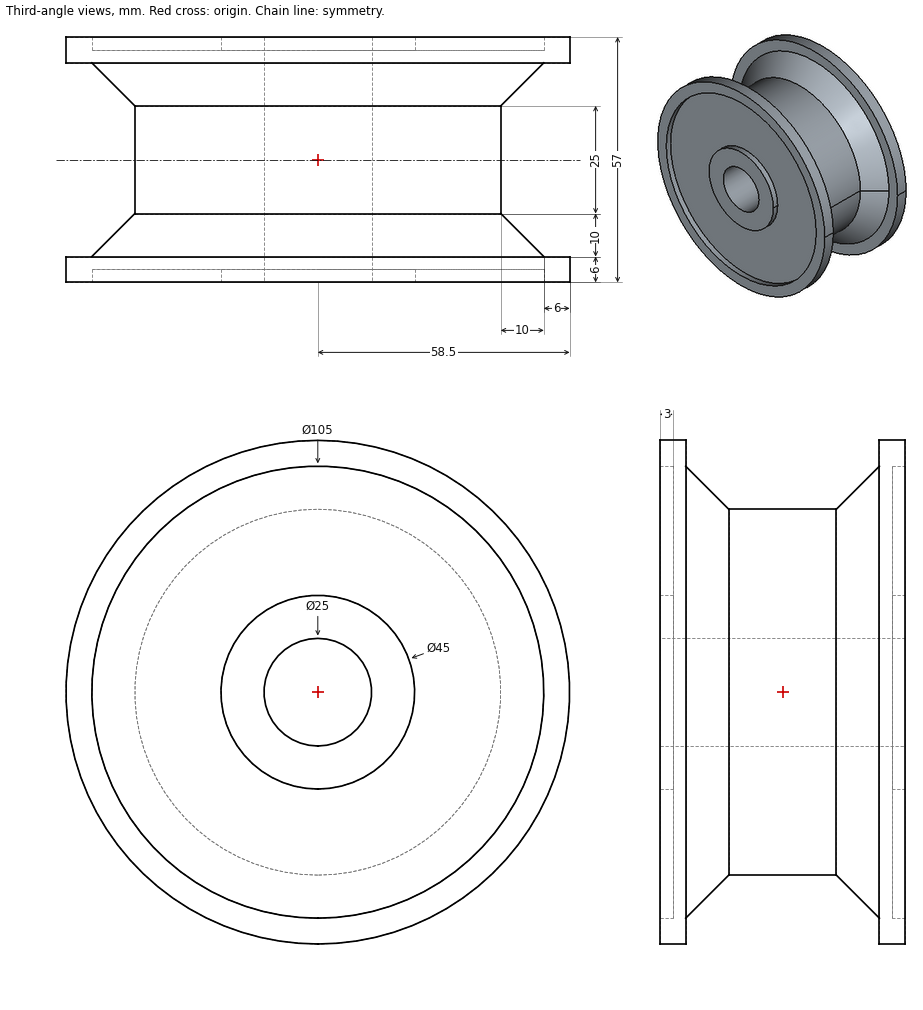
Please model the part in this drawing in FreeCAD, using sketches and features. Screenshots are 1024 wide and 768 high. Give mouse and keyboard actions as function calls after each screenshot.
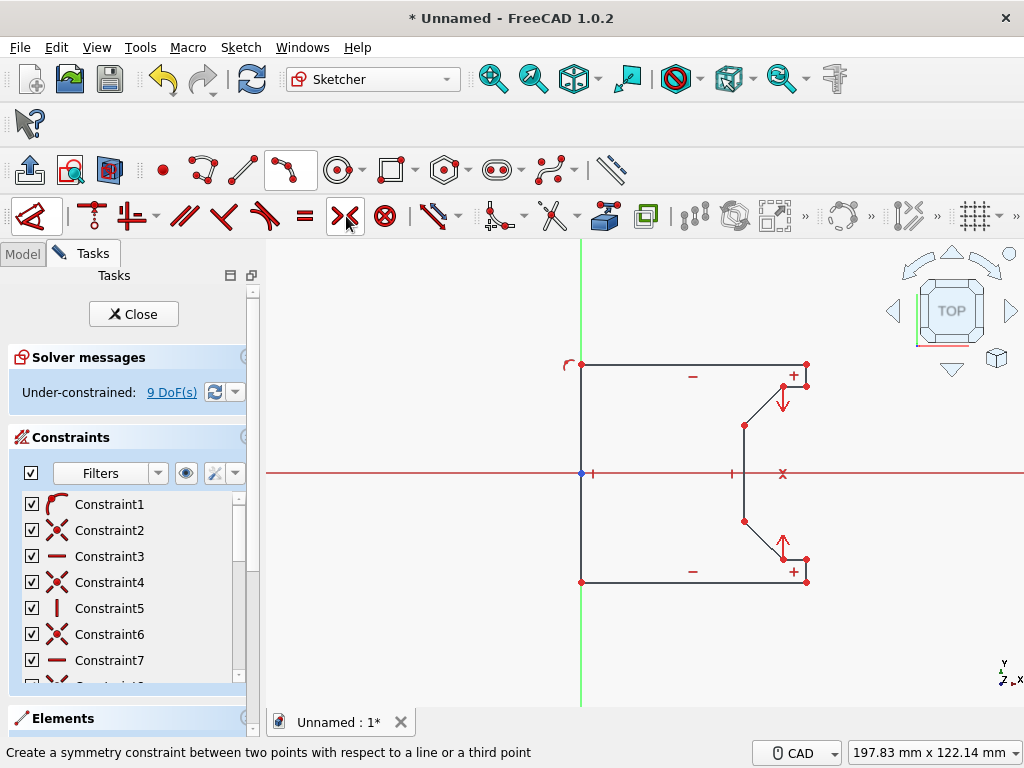
click(806, 583)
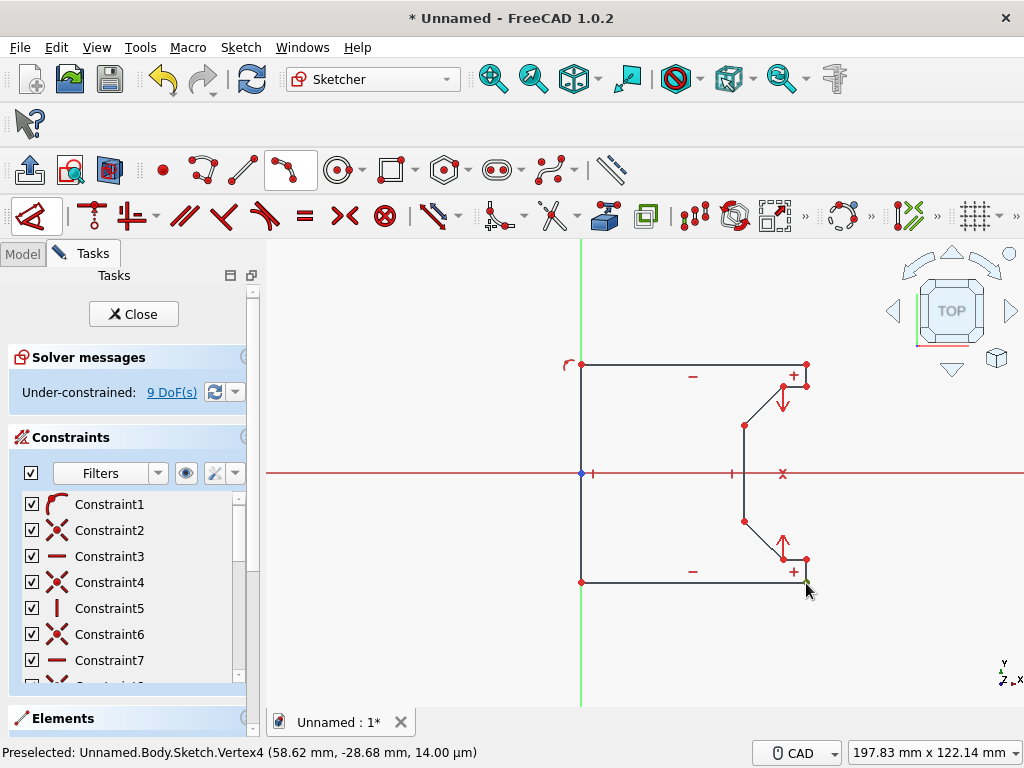
click(806, 365)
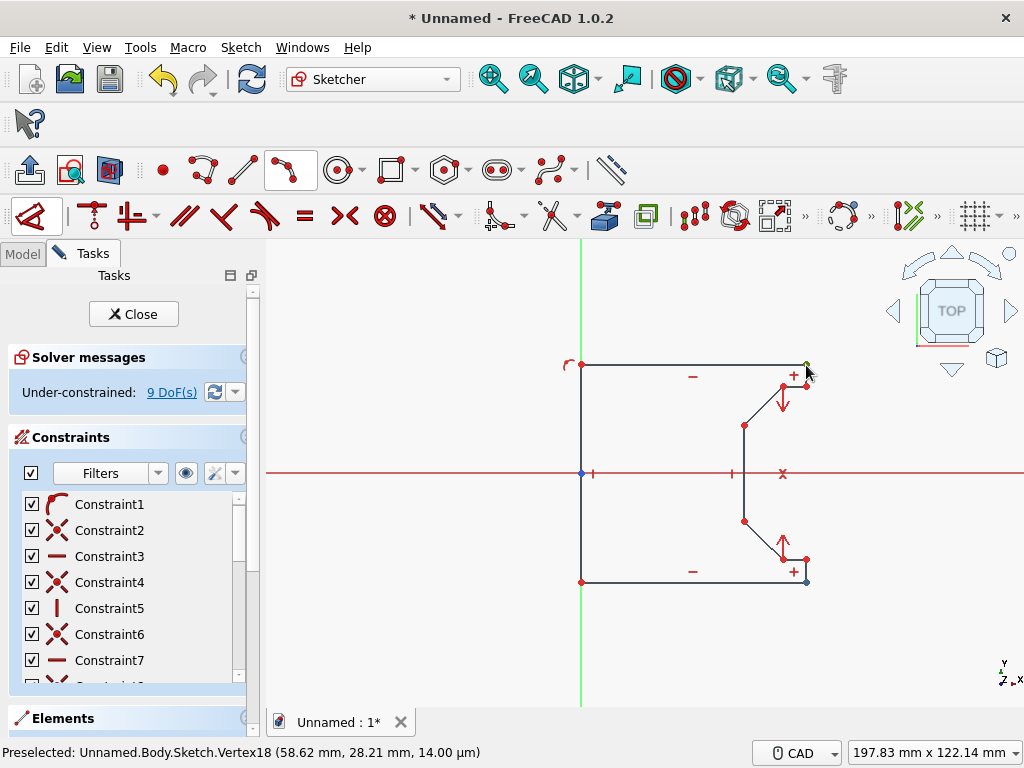
click(334, 473)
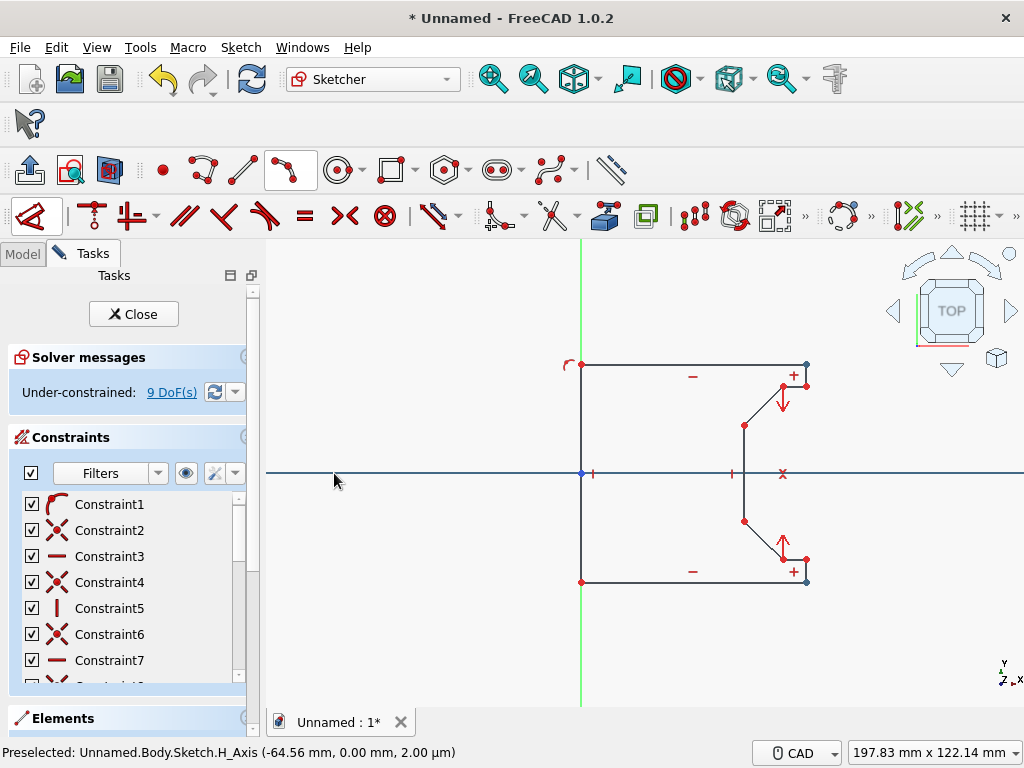
click(346, 216)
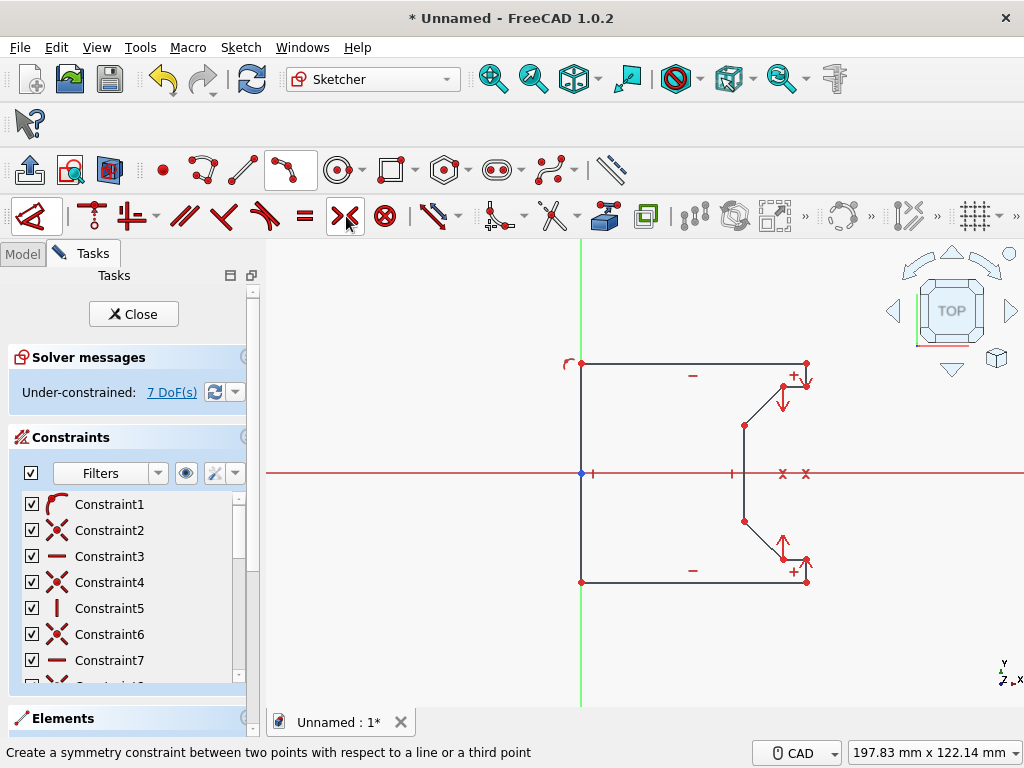
click(30, 216)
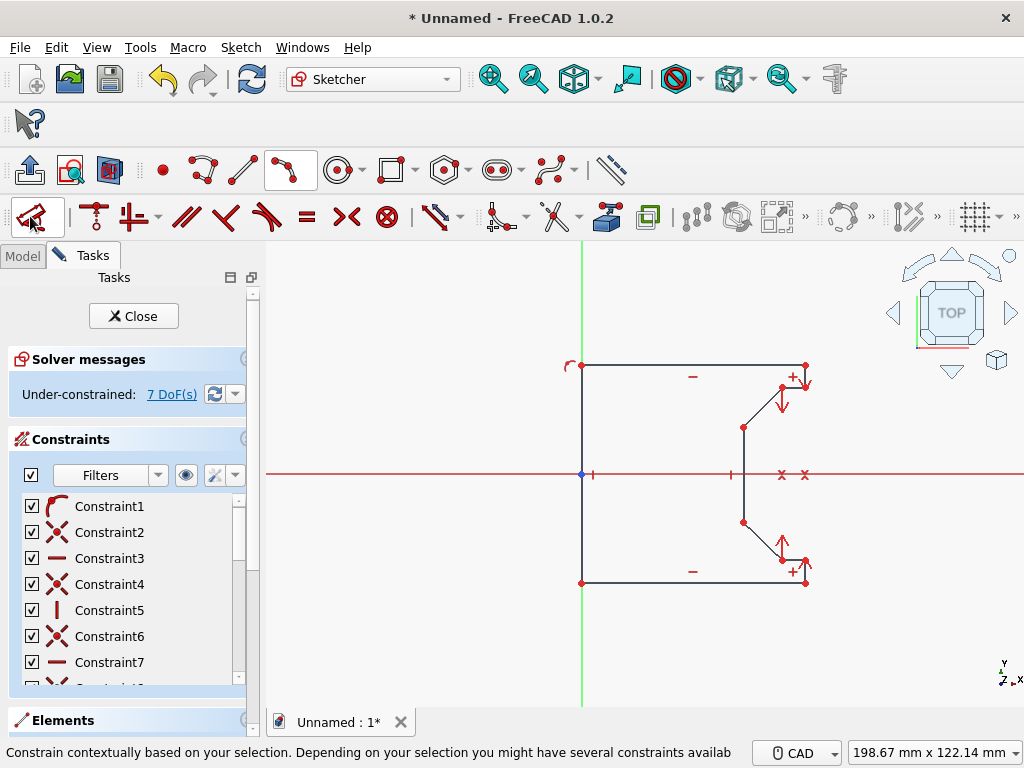
scroll(805, 574, up, 3)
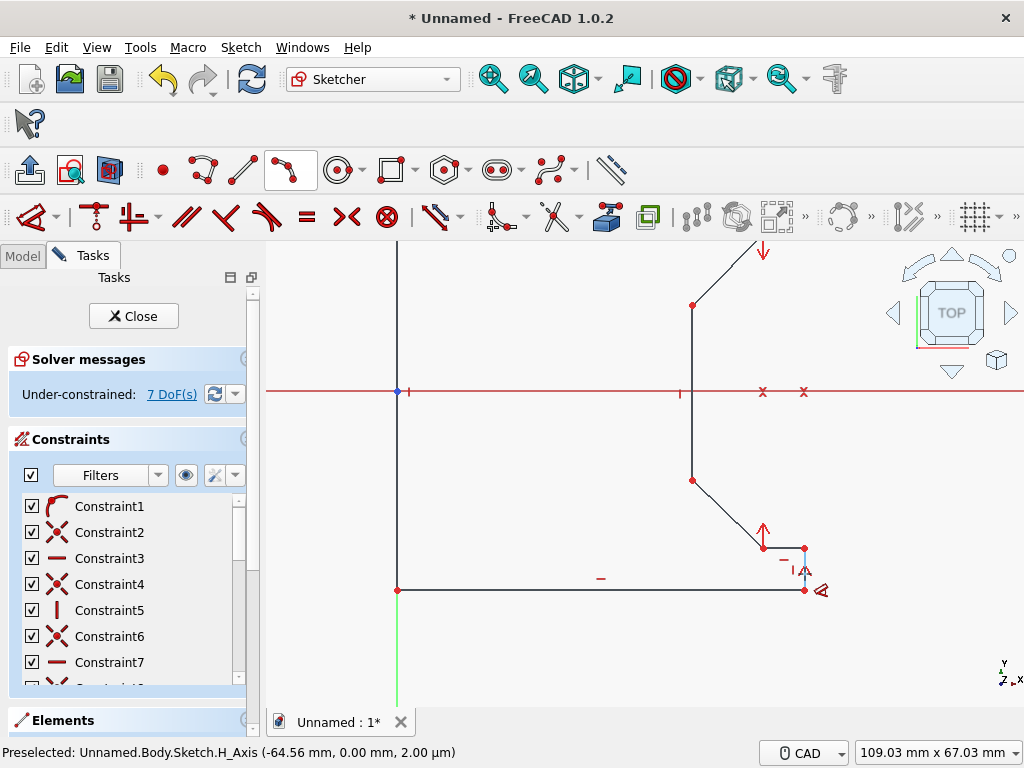
click(805, 573)
click(839, 569)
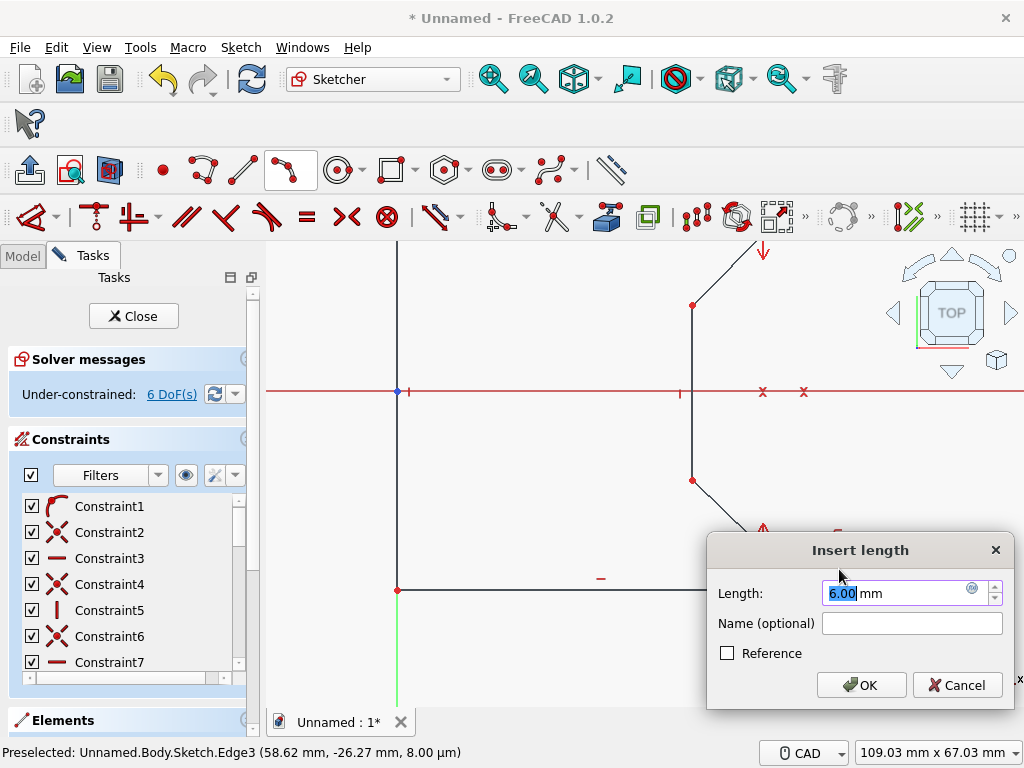
text(6)
key(Return)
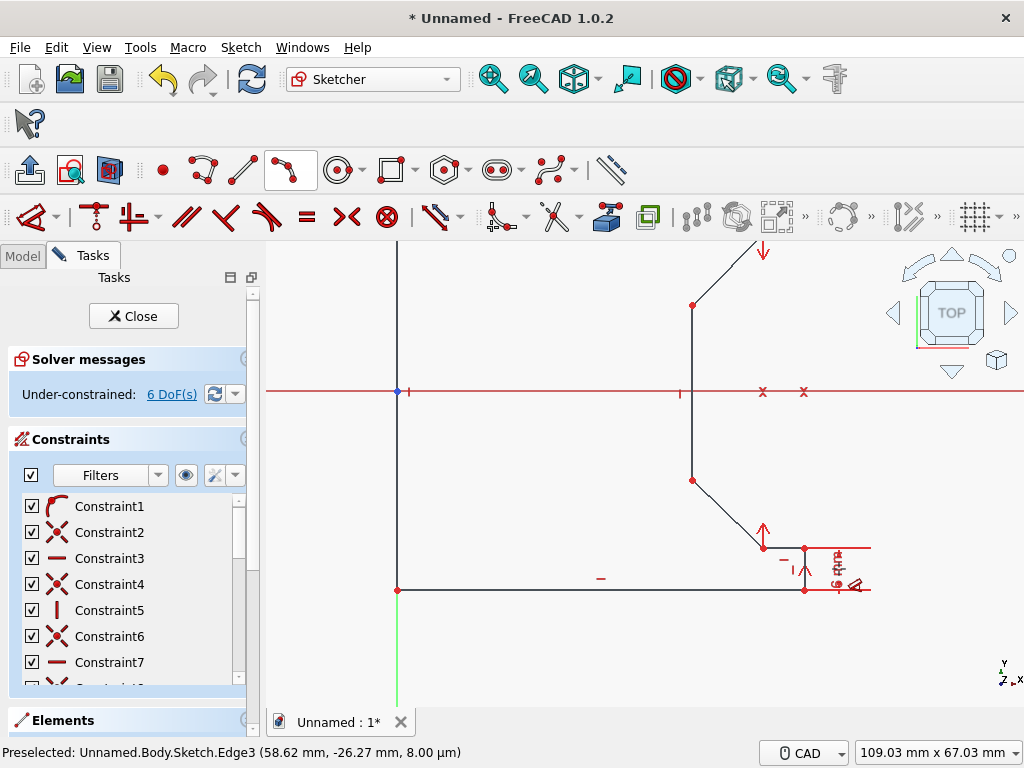
click(792, 548)
click(784, 514)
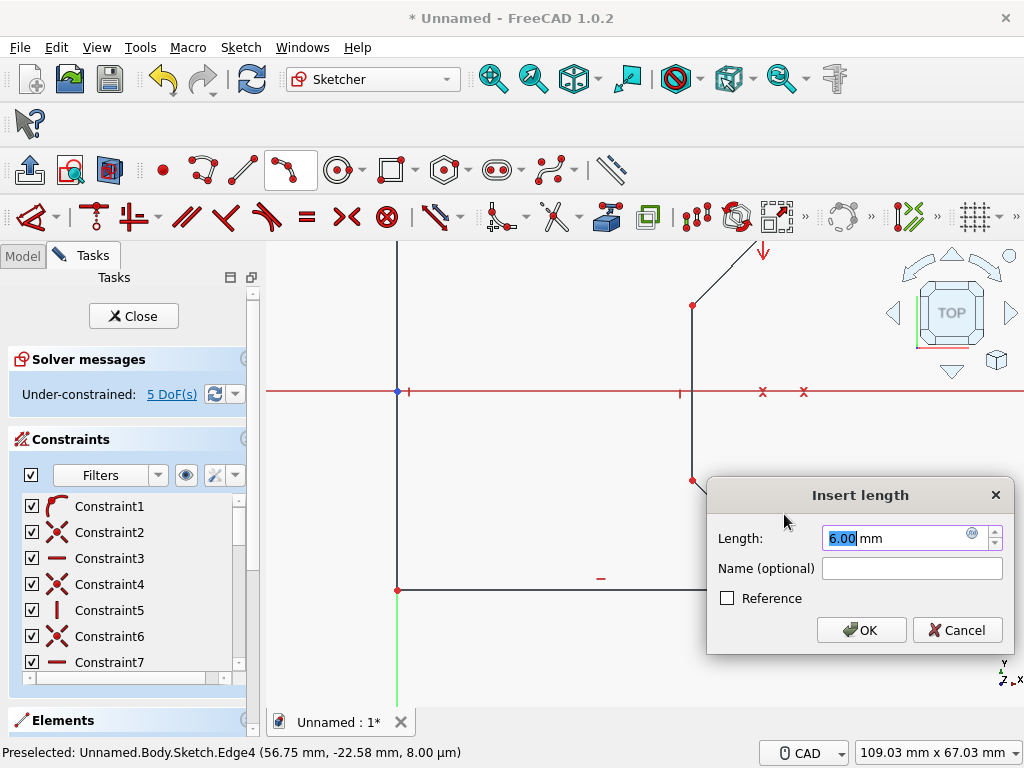
text(6)
key(Return)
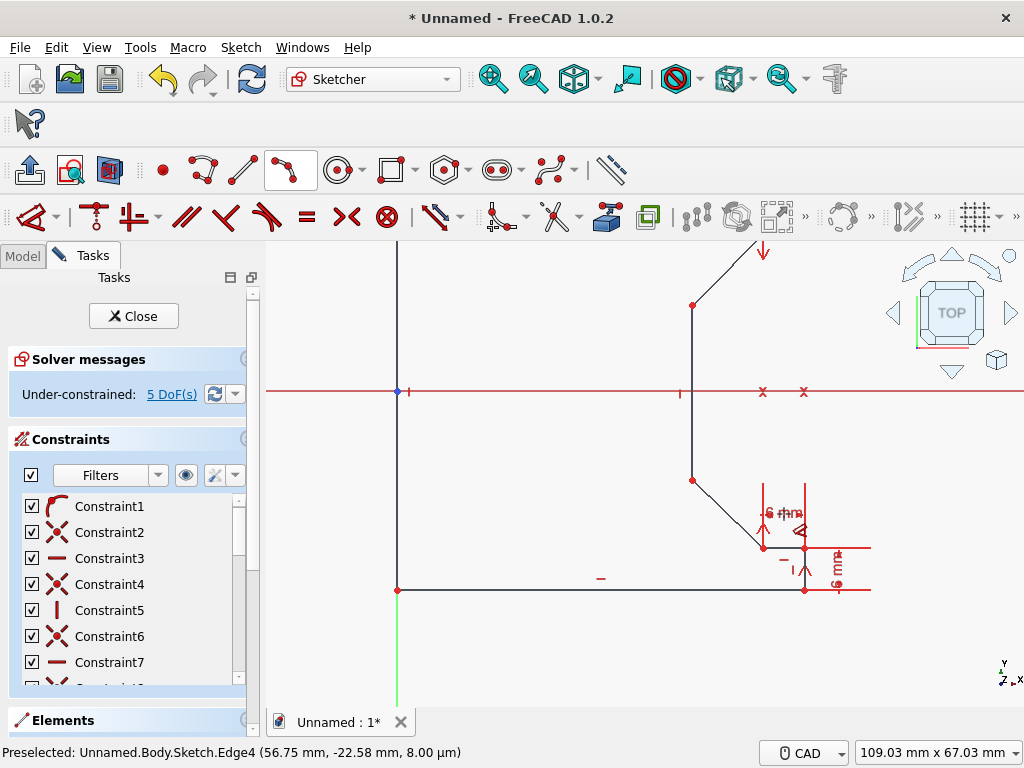
click(397, 312)
click(363, 430)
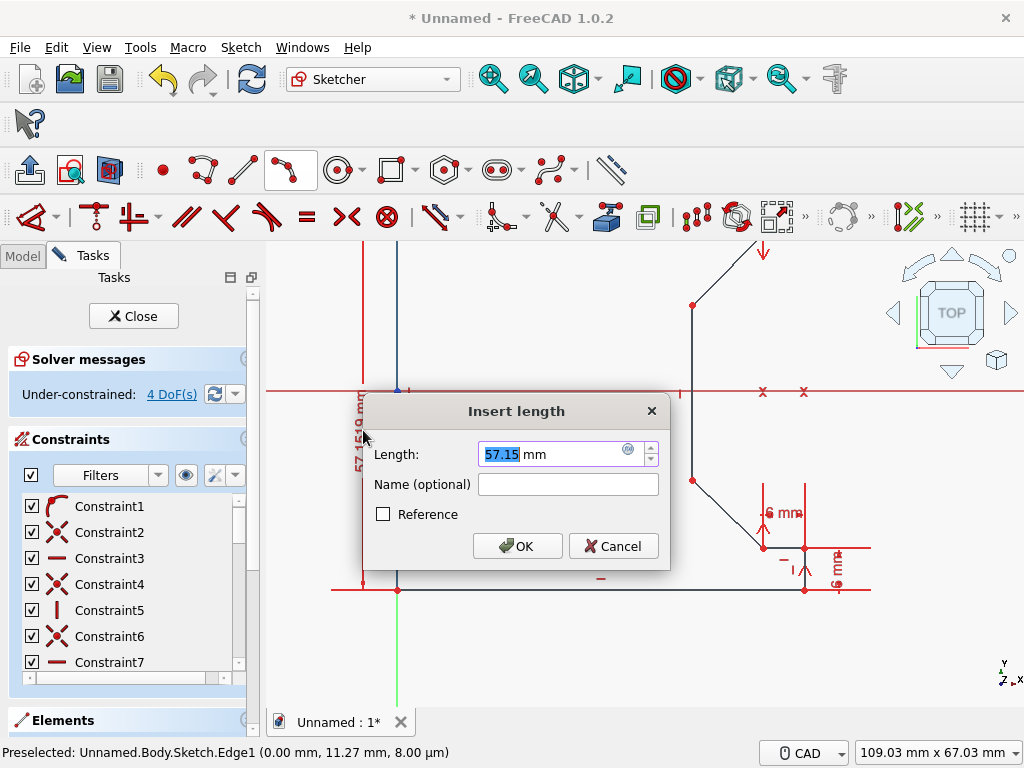
text(57)
key(Return)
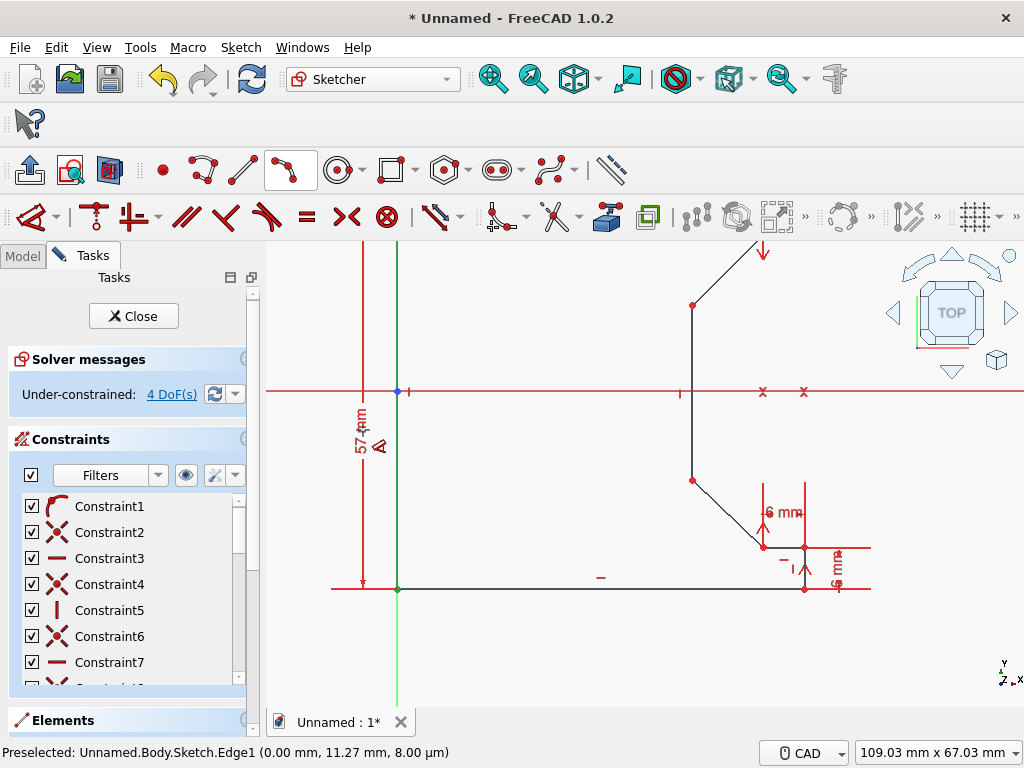
click(692, 428)
click(726, 353)